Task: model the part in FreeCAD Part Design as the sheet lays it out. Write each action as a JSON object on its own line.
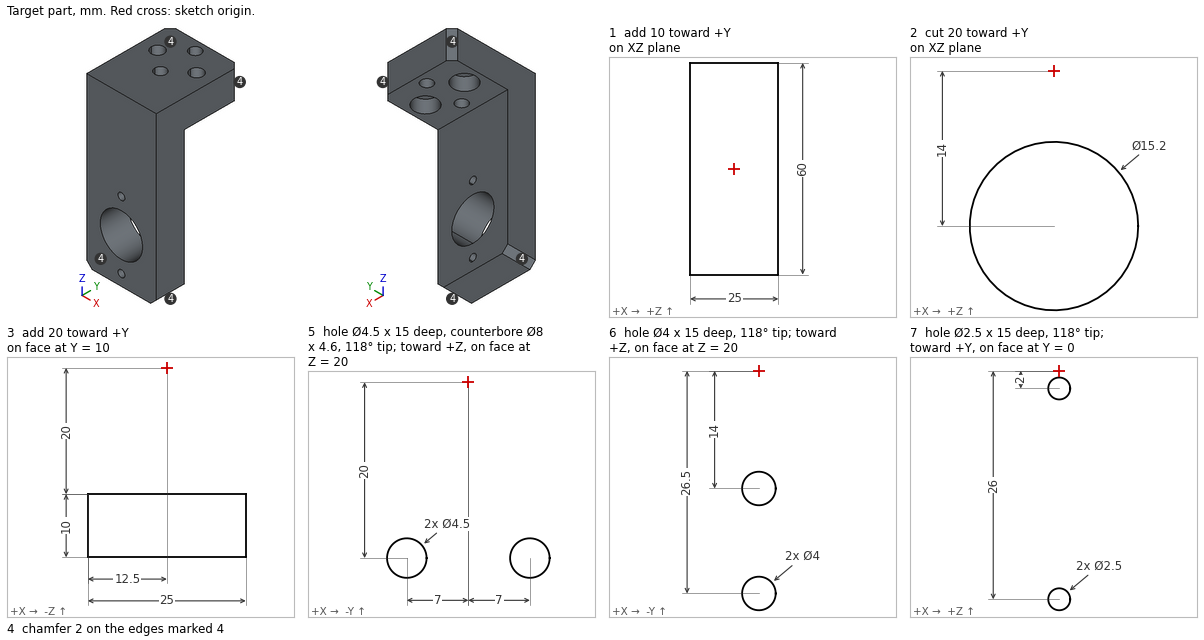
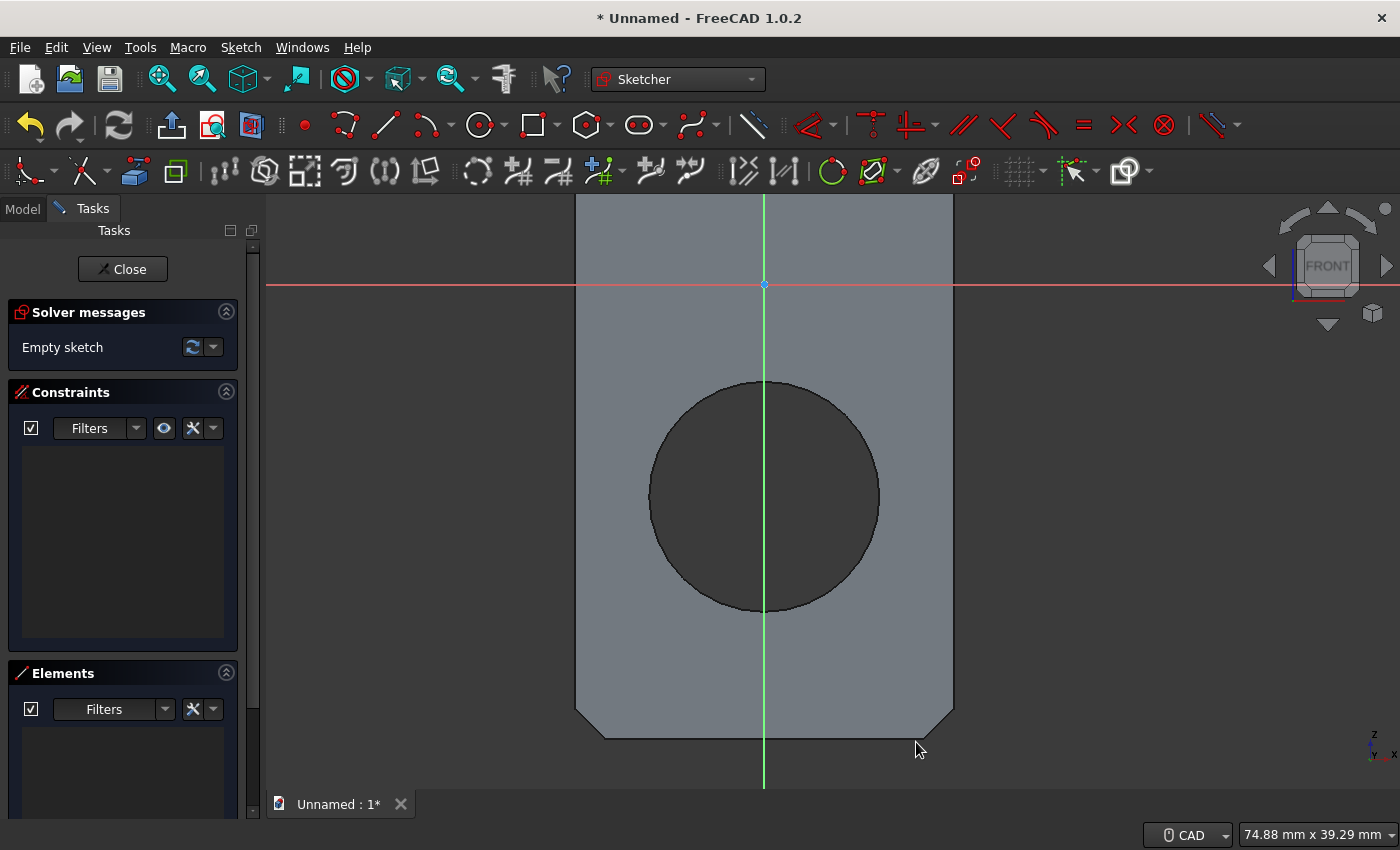
{"action": "left_click", "coordinate": [480, 126]}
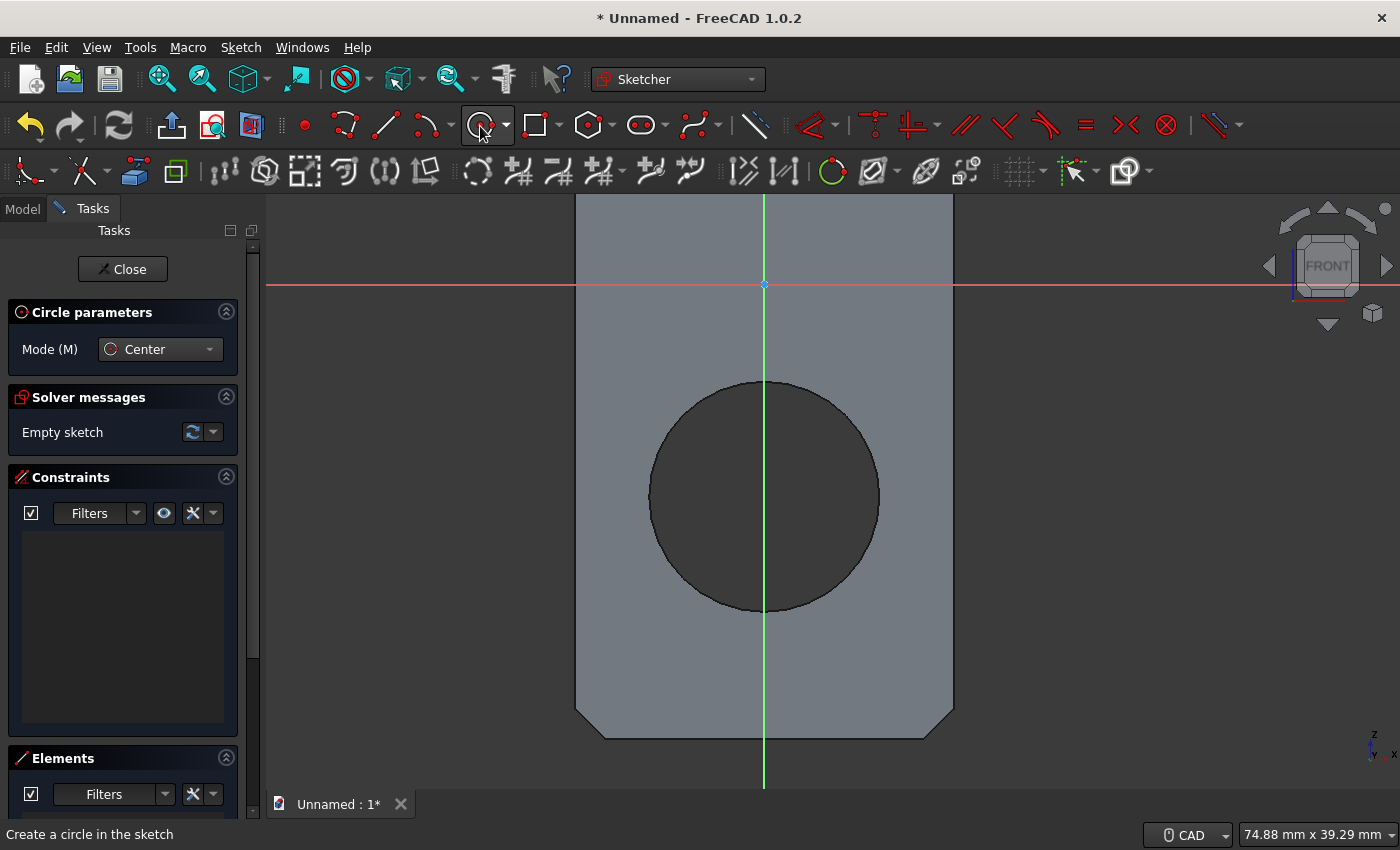
{"action": "left_click", "coordinate": [764, 679]}
{"action": "left_click", "coordinate": [782, 672]}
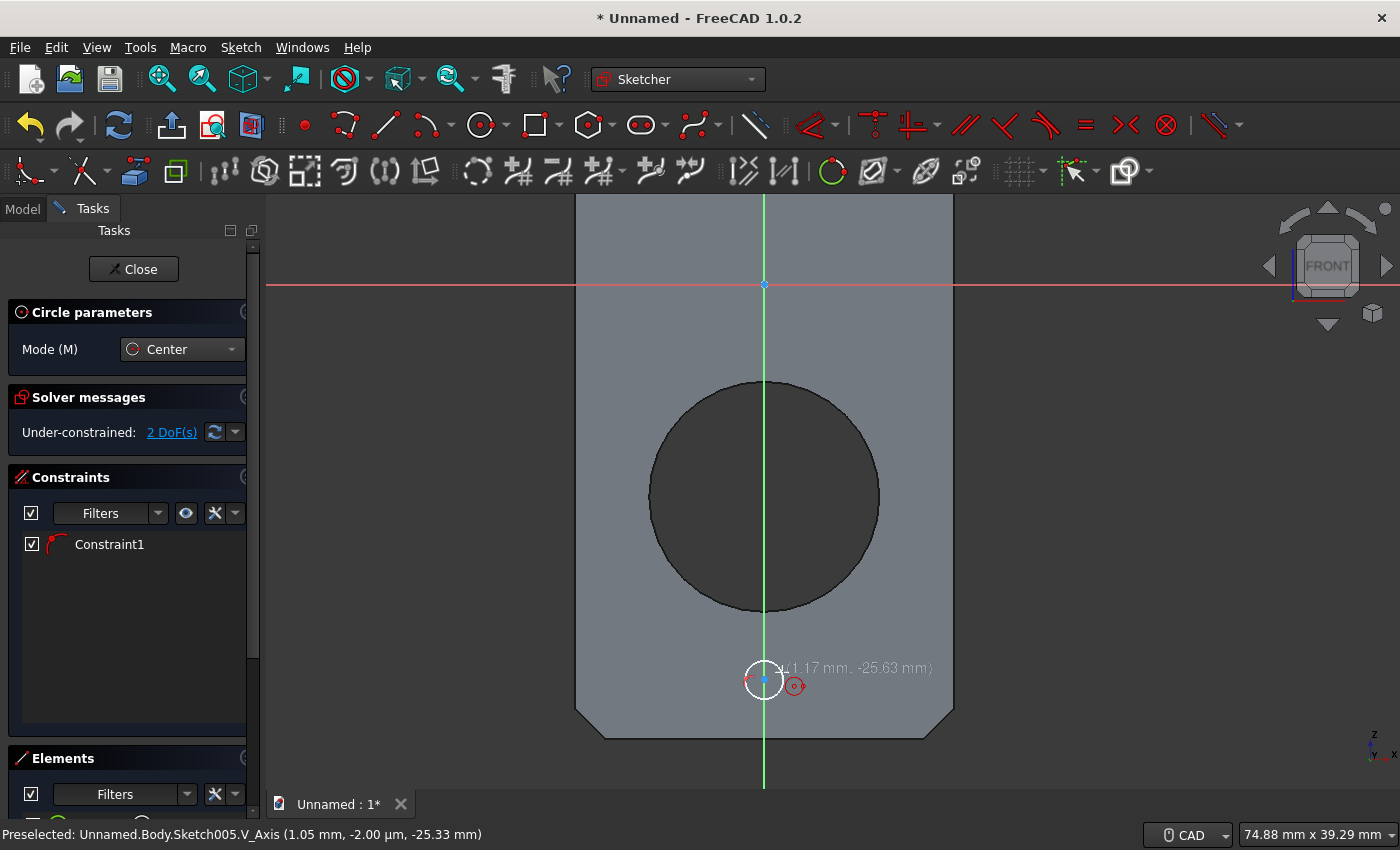
{"action": "left_click", "coordinate": [764, 315]}
{"action": "left_click", "coordinate": [782, 309]}
{"action": "key", "text": "Escape"}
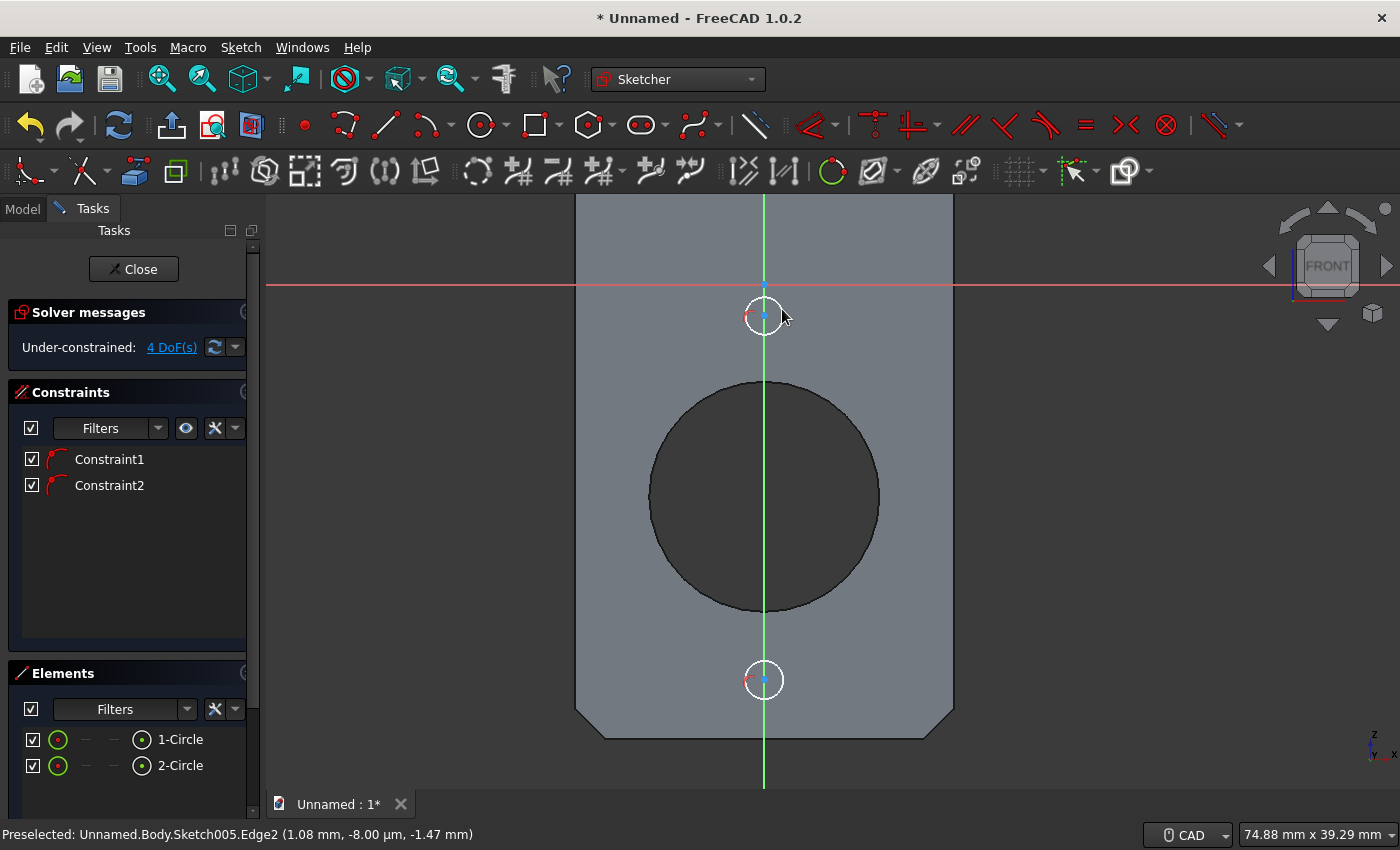
{"action": "left_click", "coordinate": [778, 666]}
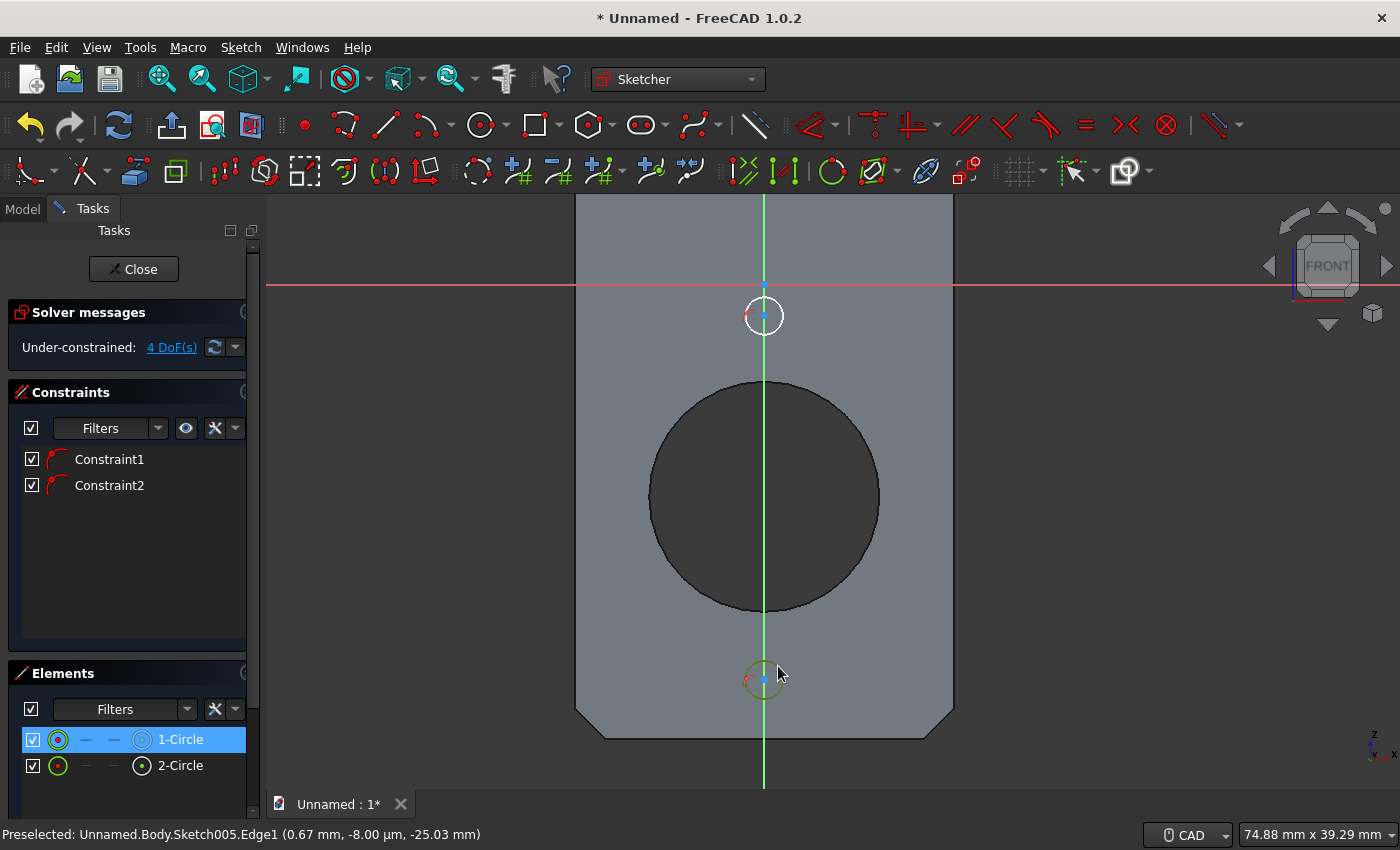
{"action": "left_click", "coordinate": [777, 303]}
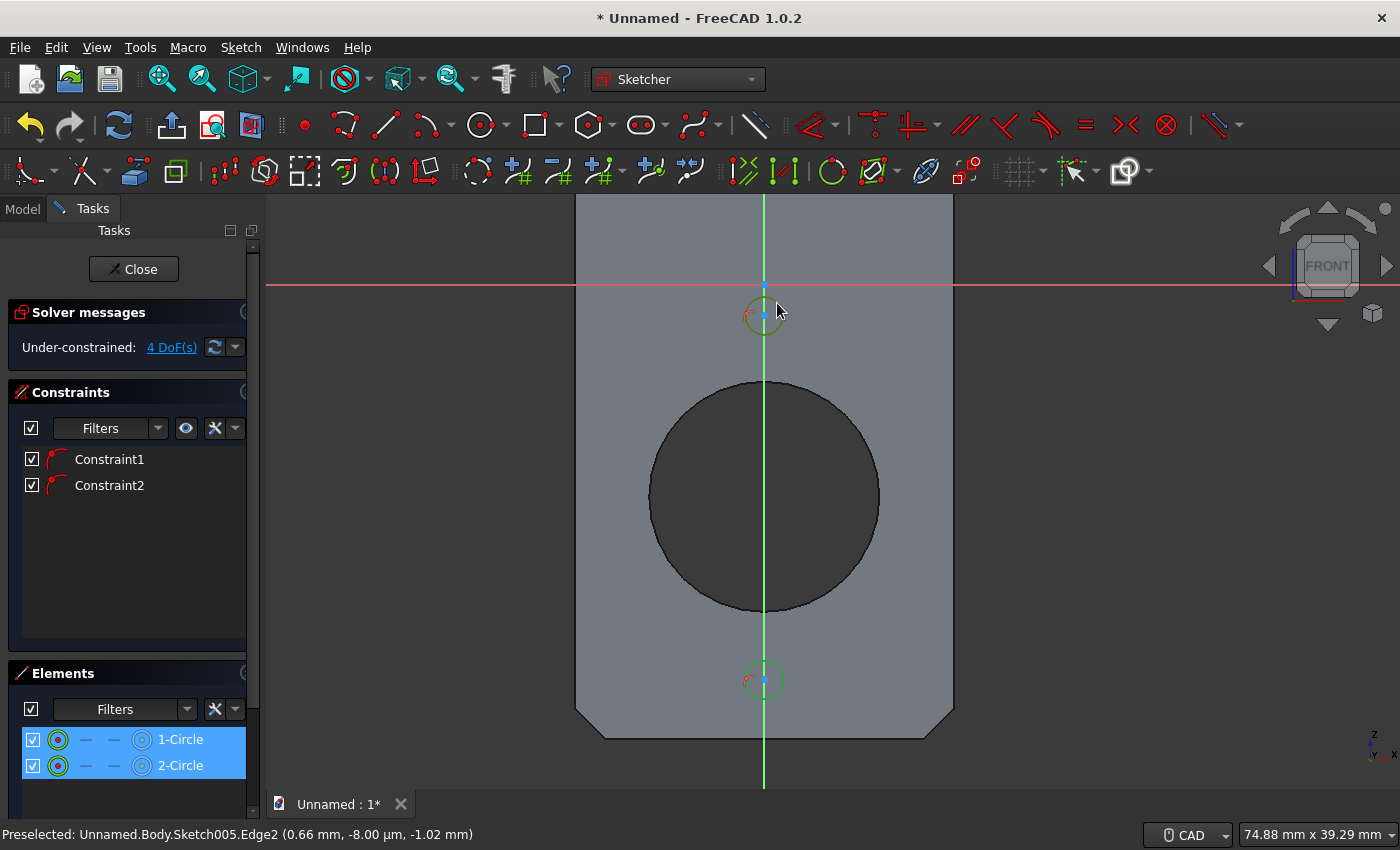
{"action": "left_click", "coordinate": [1086, 126]}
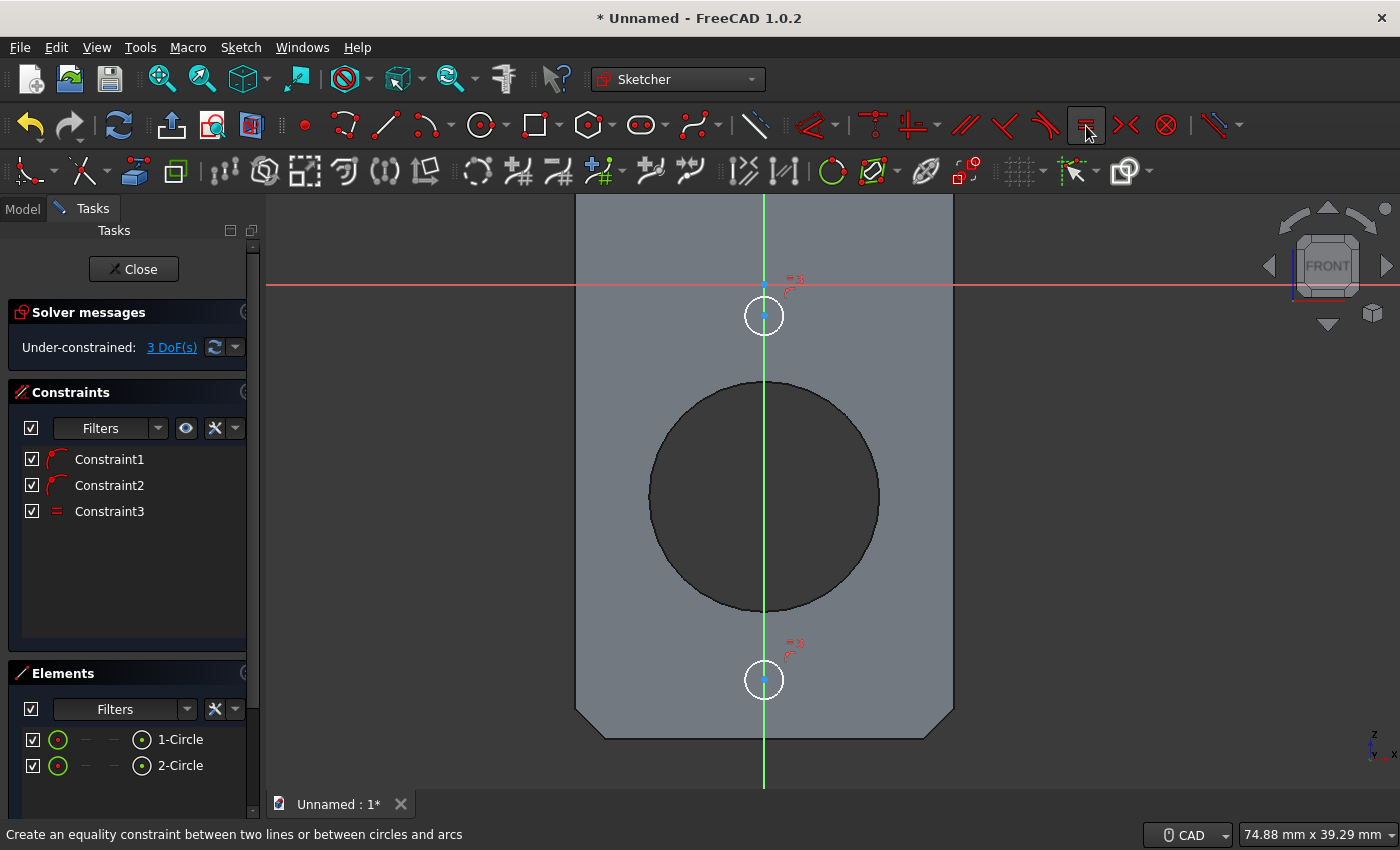
{"action": "key", "text": "d"}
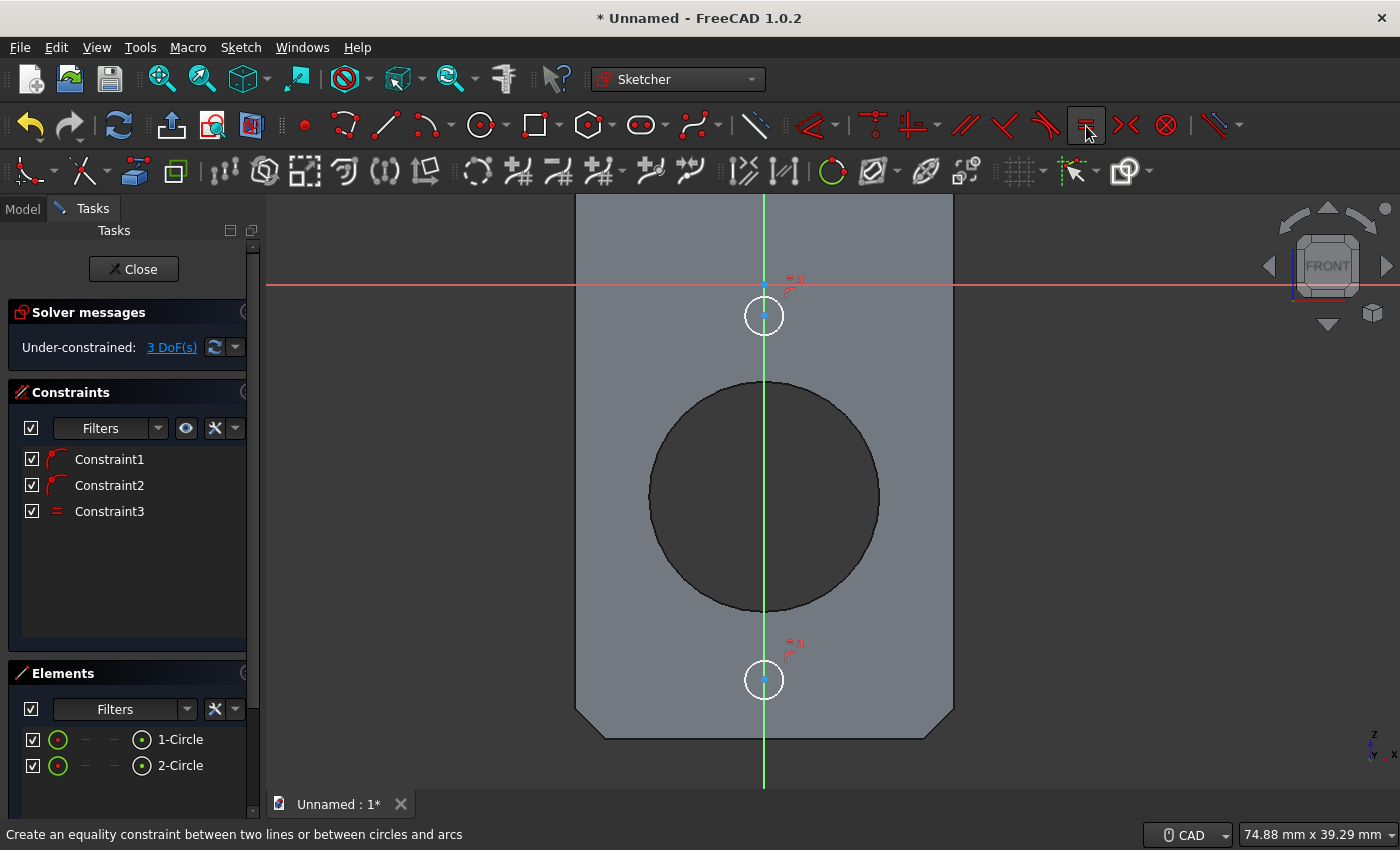
{"action": "left_click", "coordinate": [778, 666]}
{"action": "left_click", "coordinate": [800, 643]}